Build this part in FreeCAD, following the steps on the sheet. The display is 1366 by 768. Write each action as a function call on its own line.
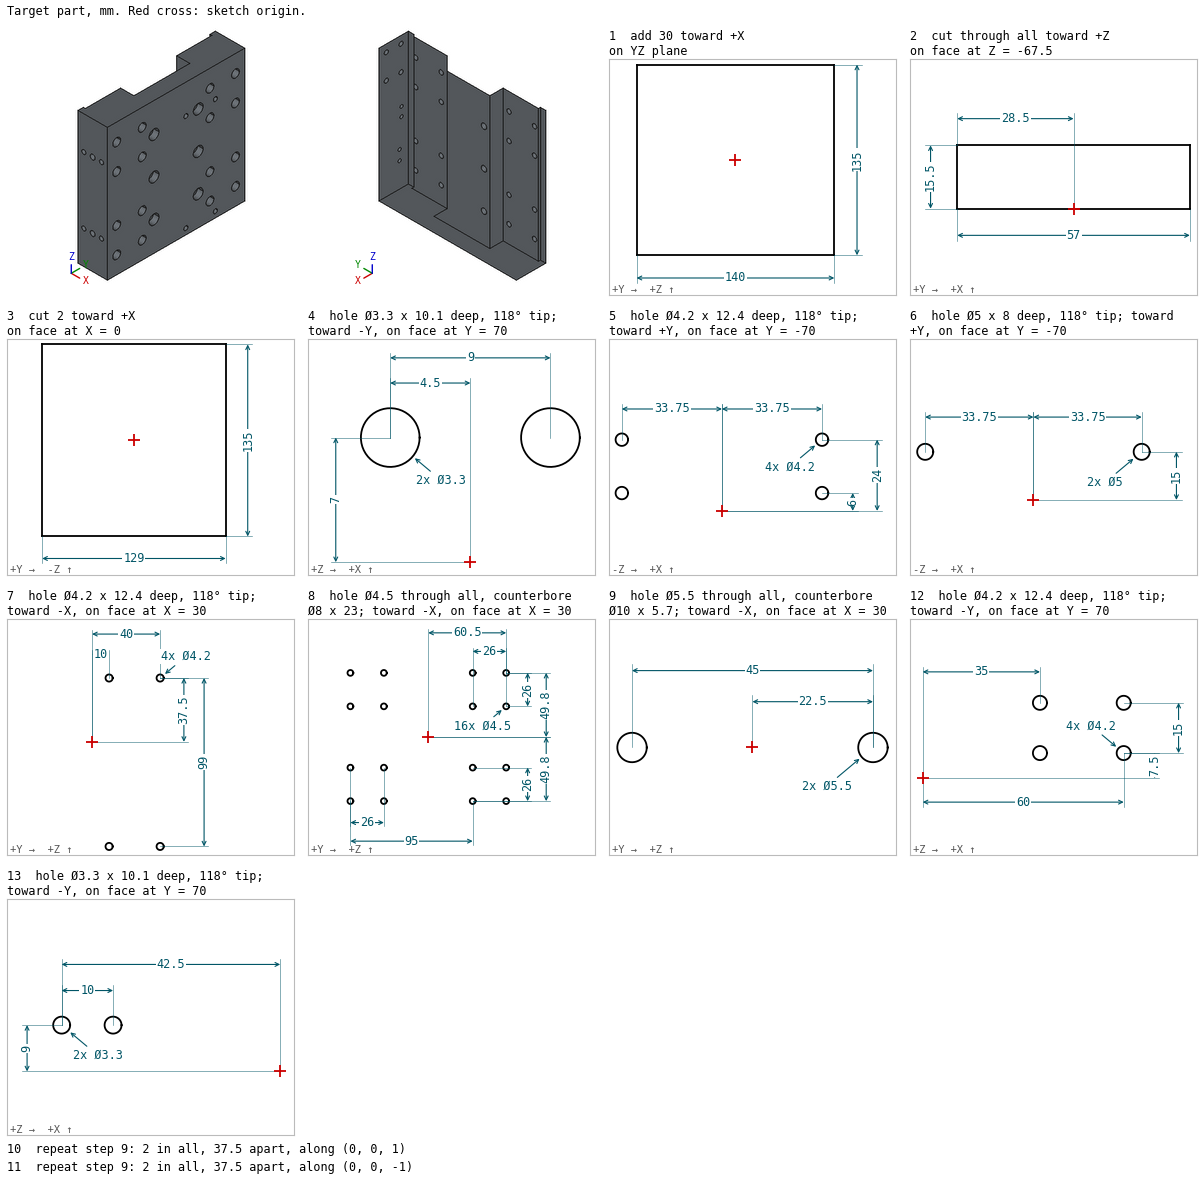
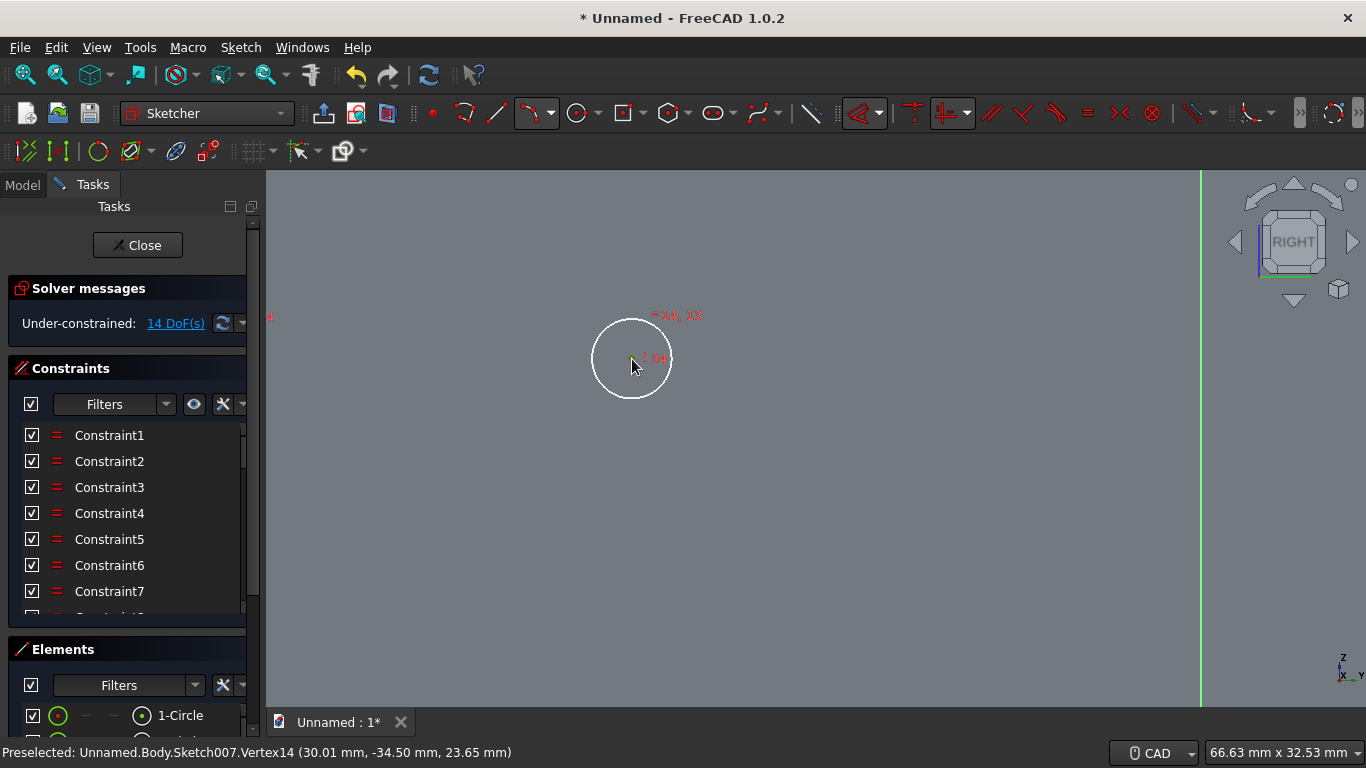
click(970, 114)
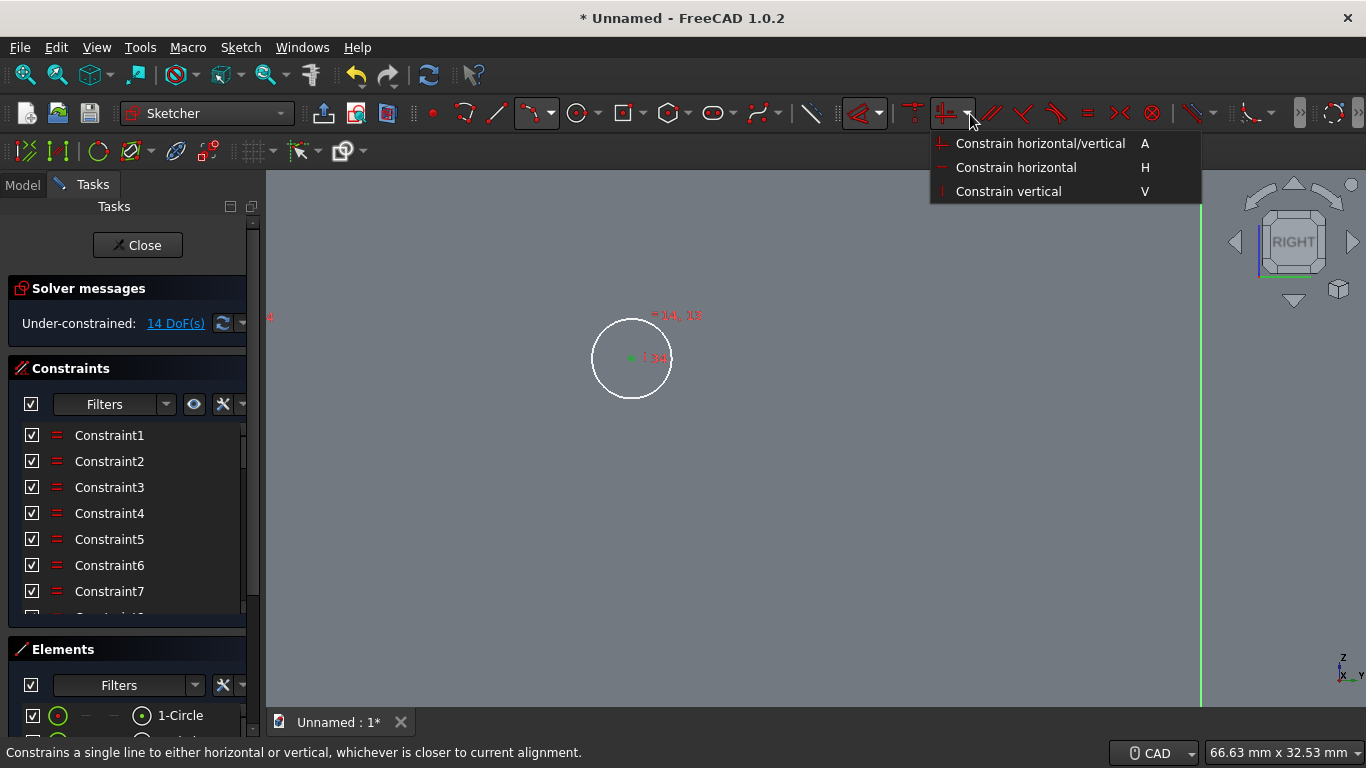
click(1066, 167)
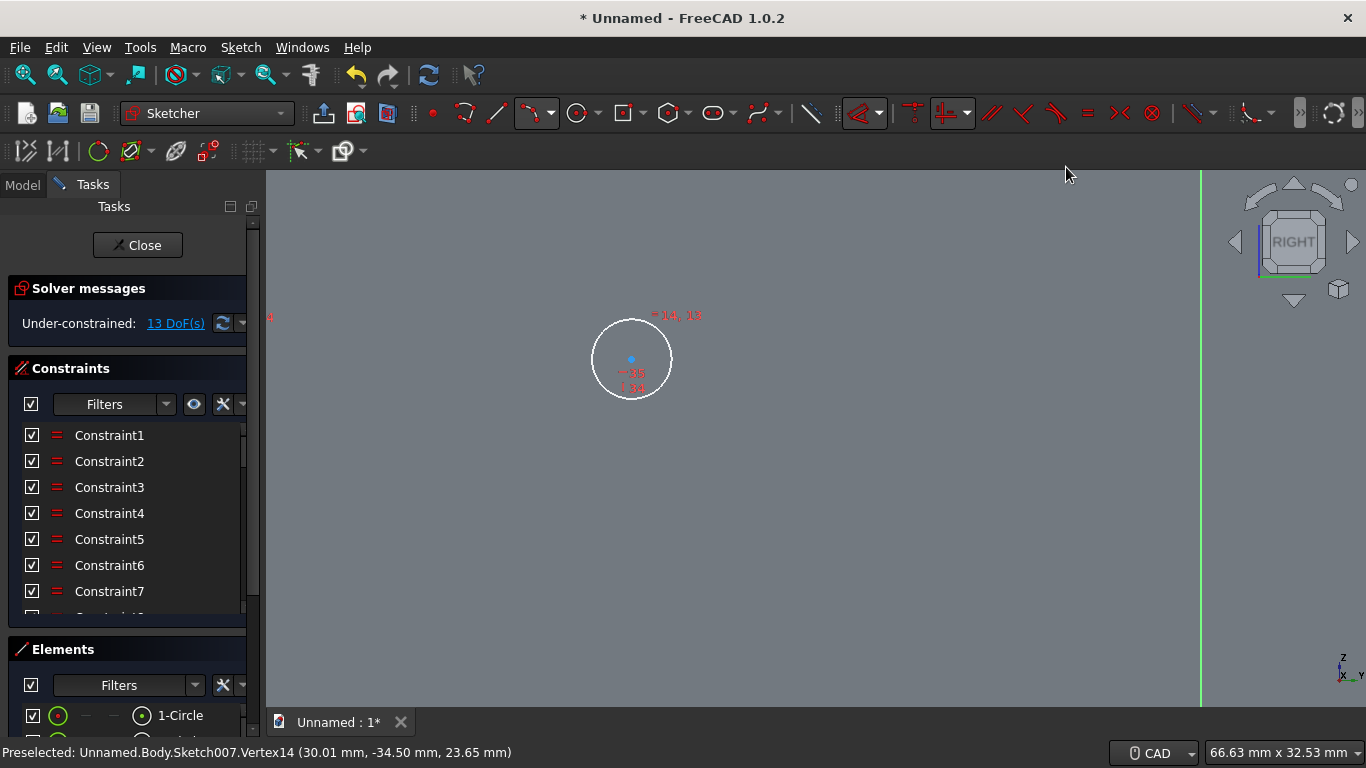
scroll(633, 360, down, 8)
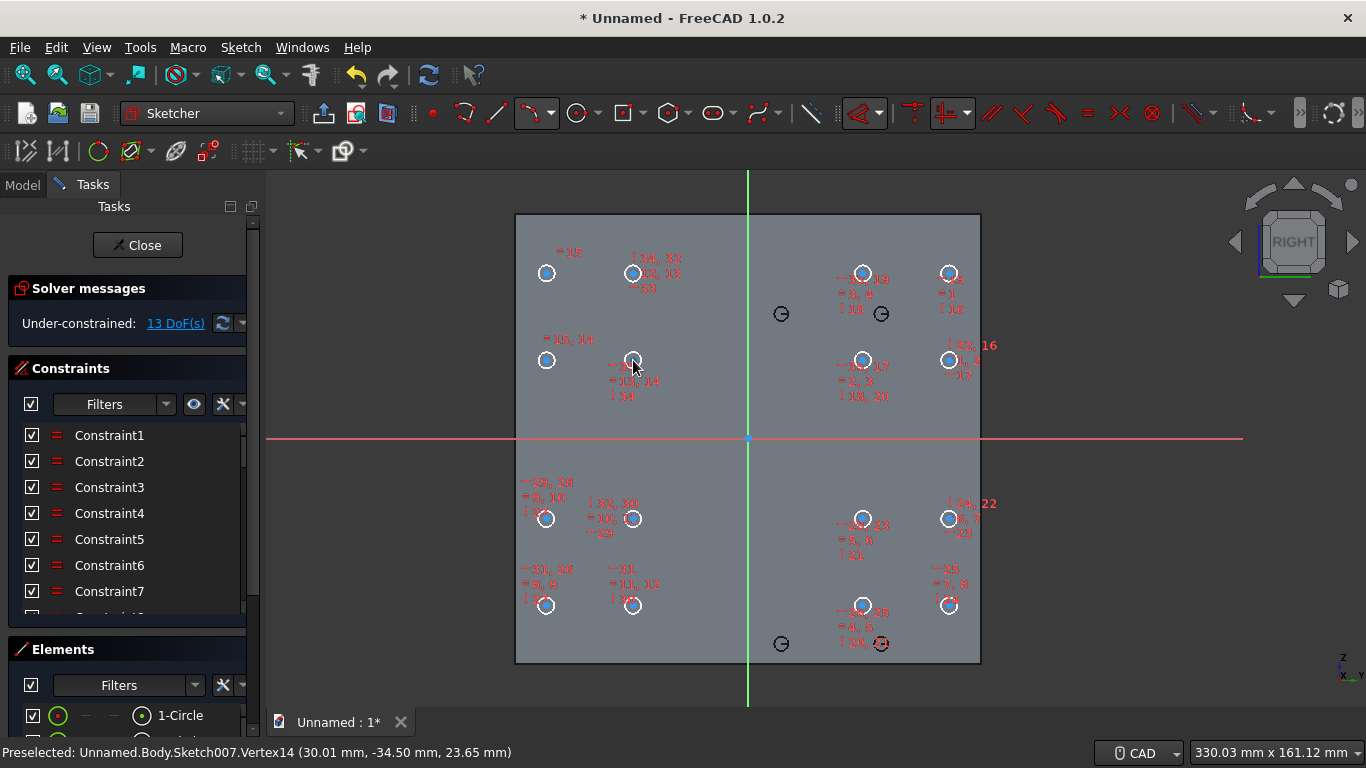
click(546, 519)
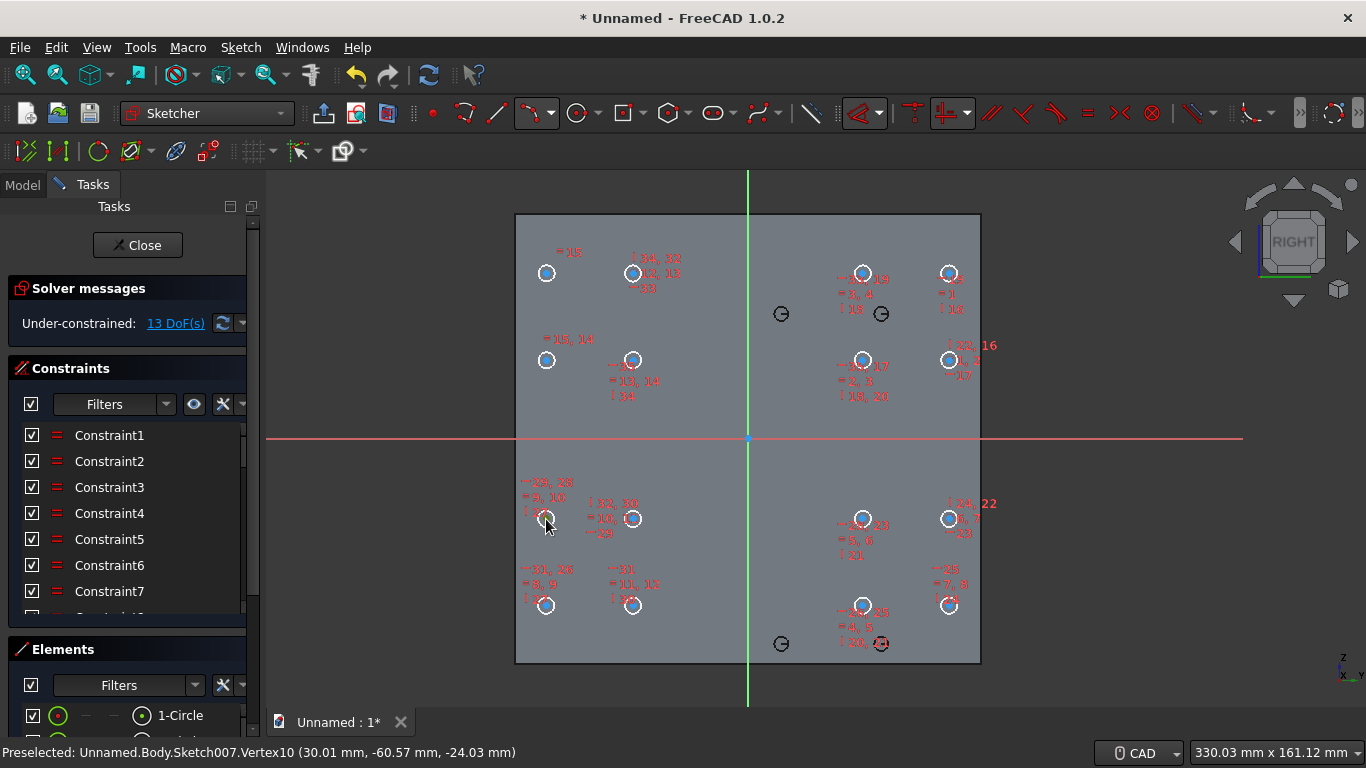
click(547, 360)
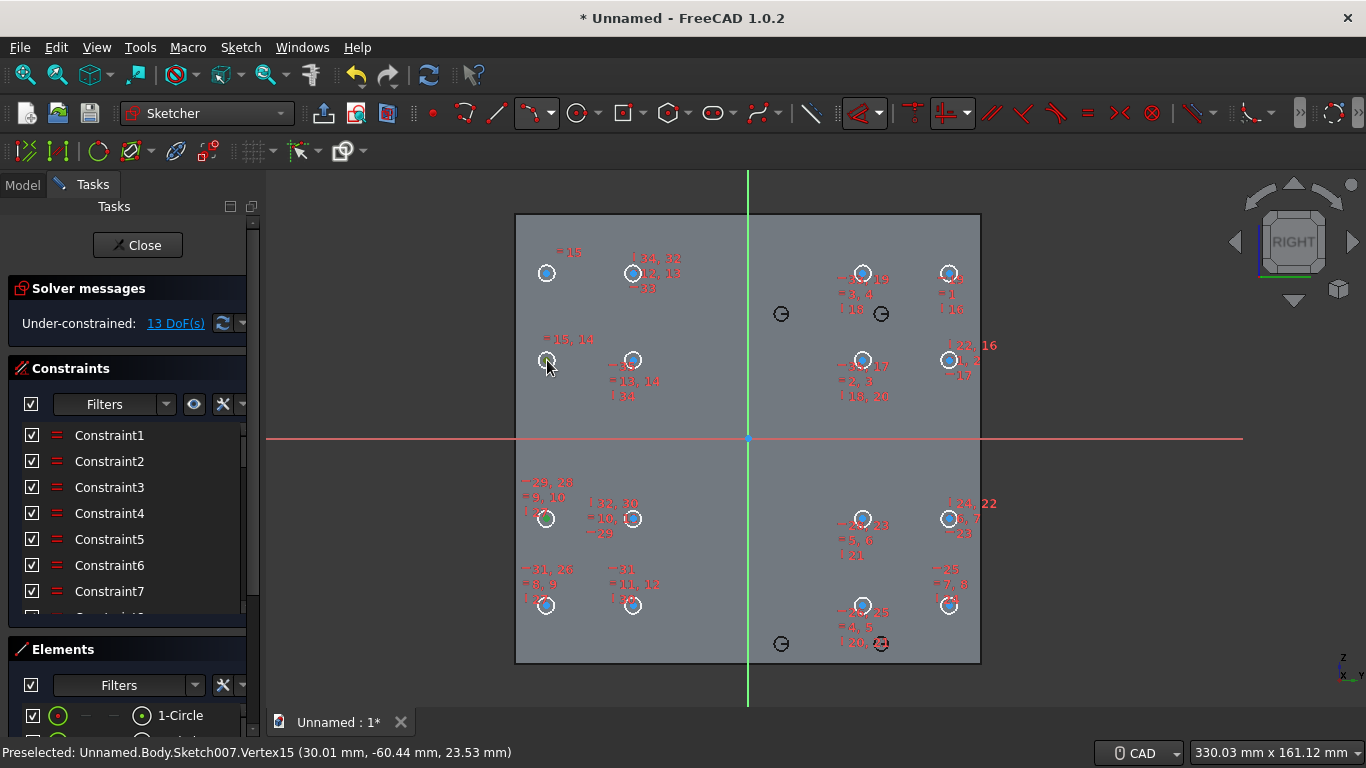
key(v)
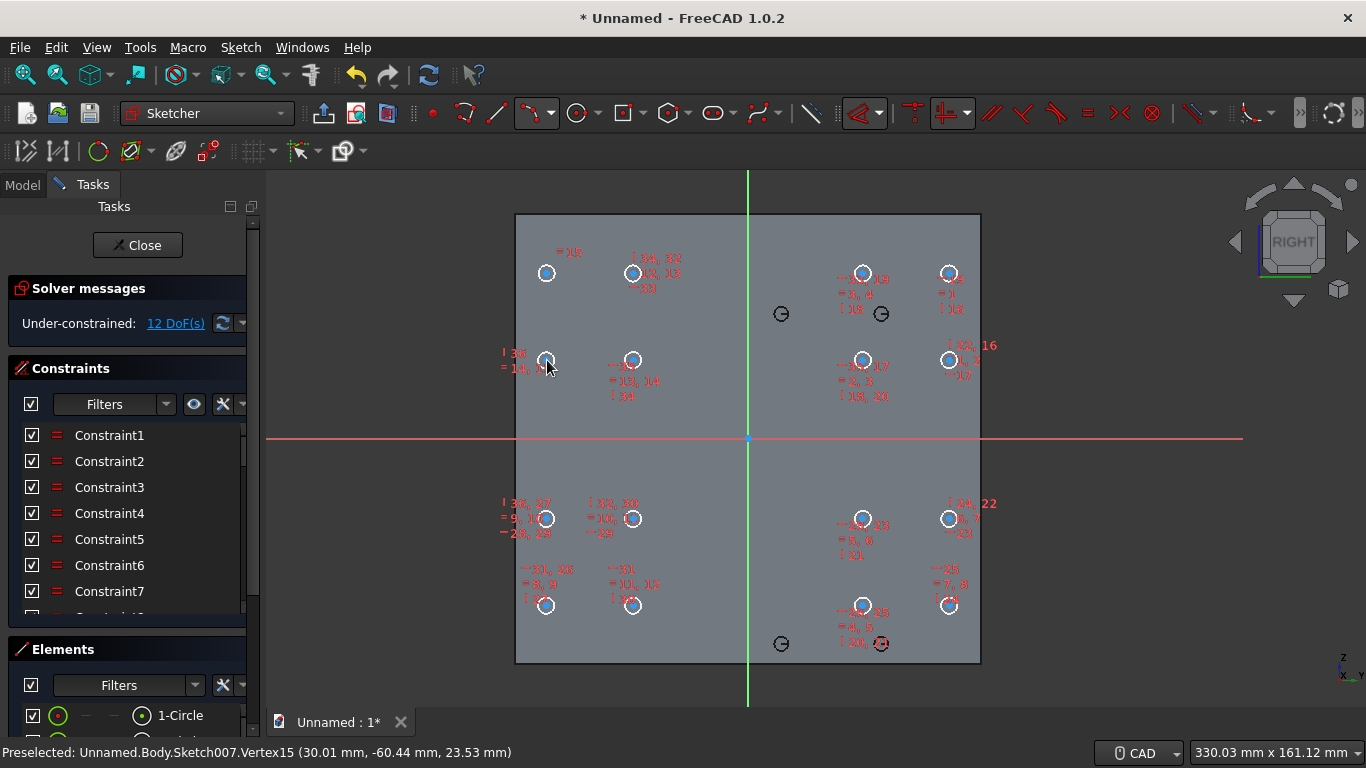
click(631, 358)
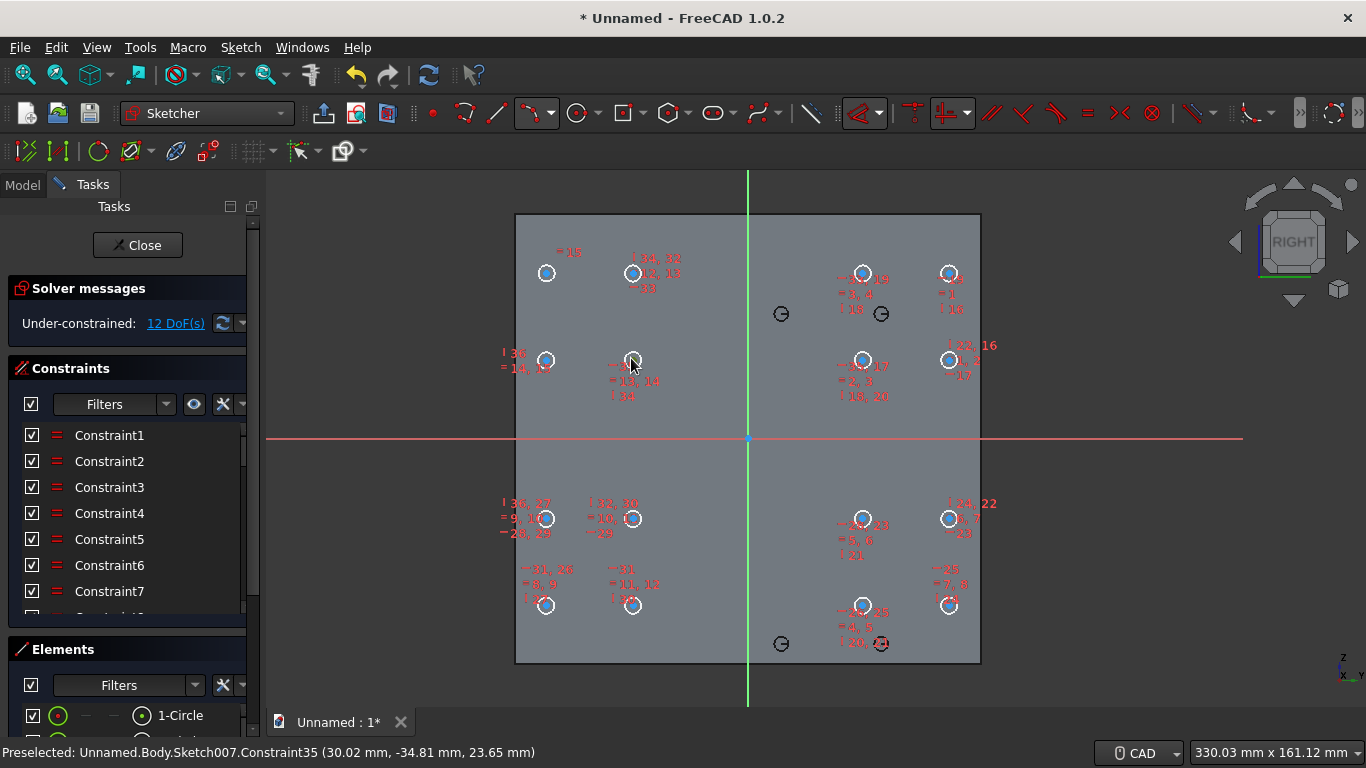
scroll(546, 360, up, 4)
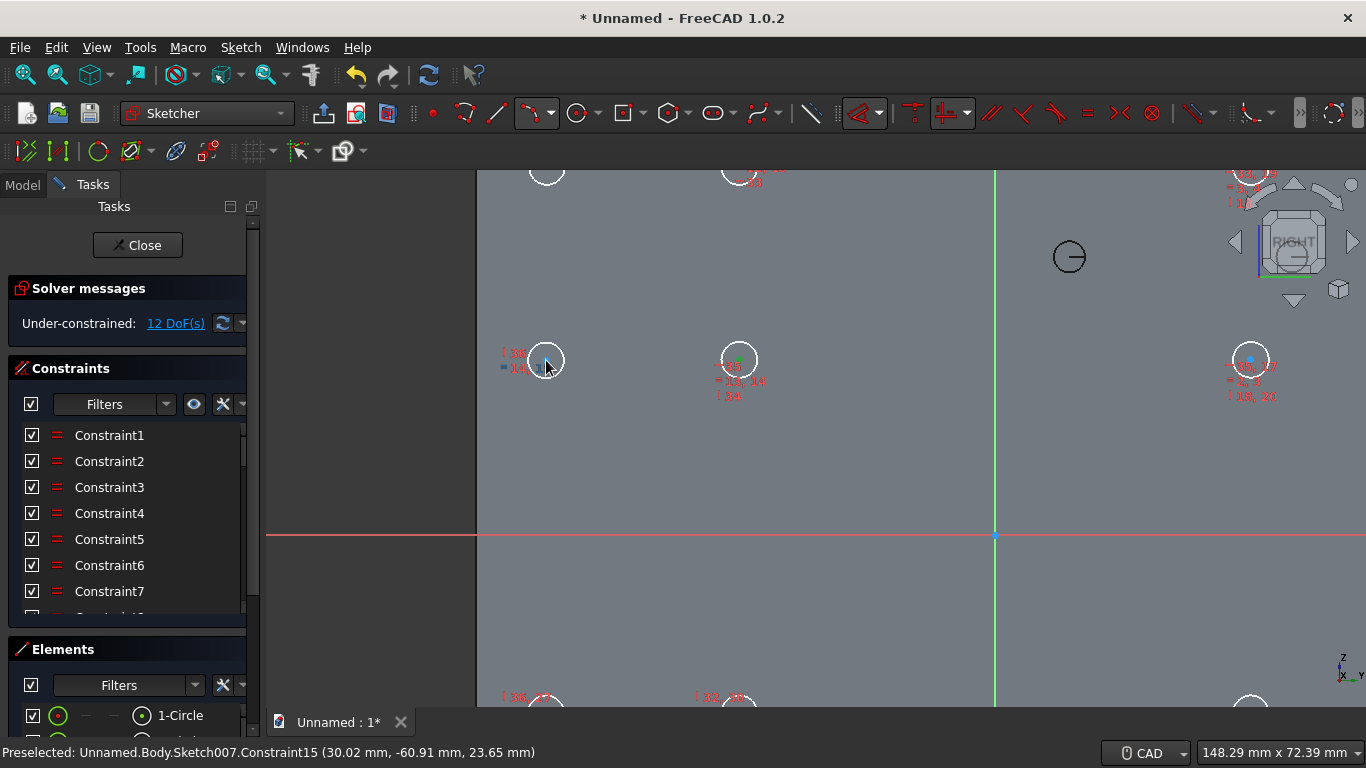
scroll(546, 360, up, 4)